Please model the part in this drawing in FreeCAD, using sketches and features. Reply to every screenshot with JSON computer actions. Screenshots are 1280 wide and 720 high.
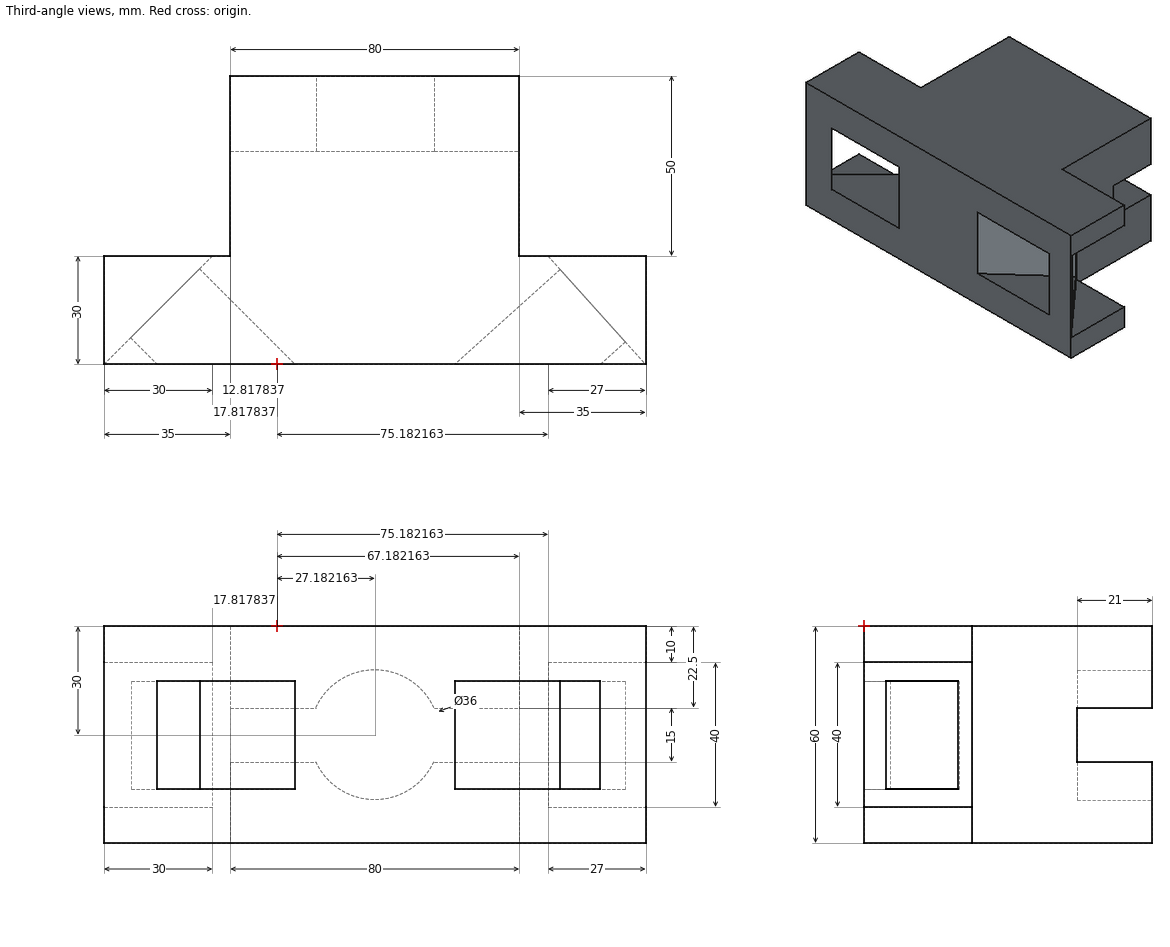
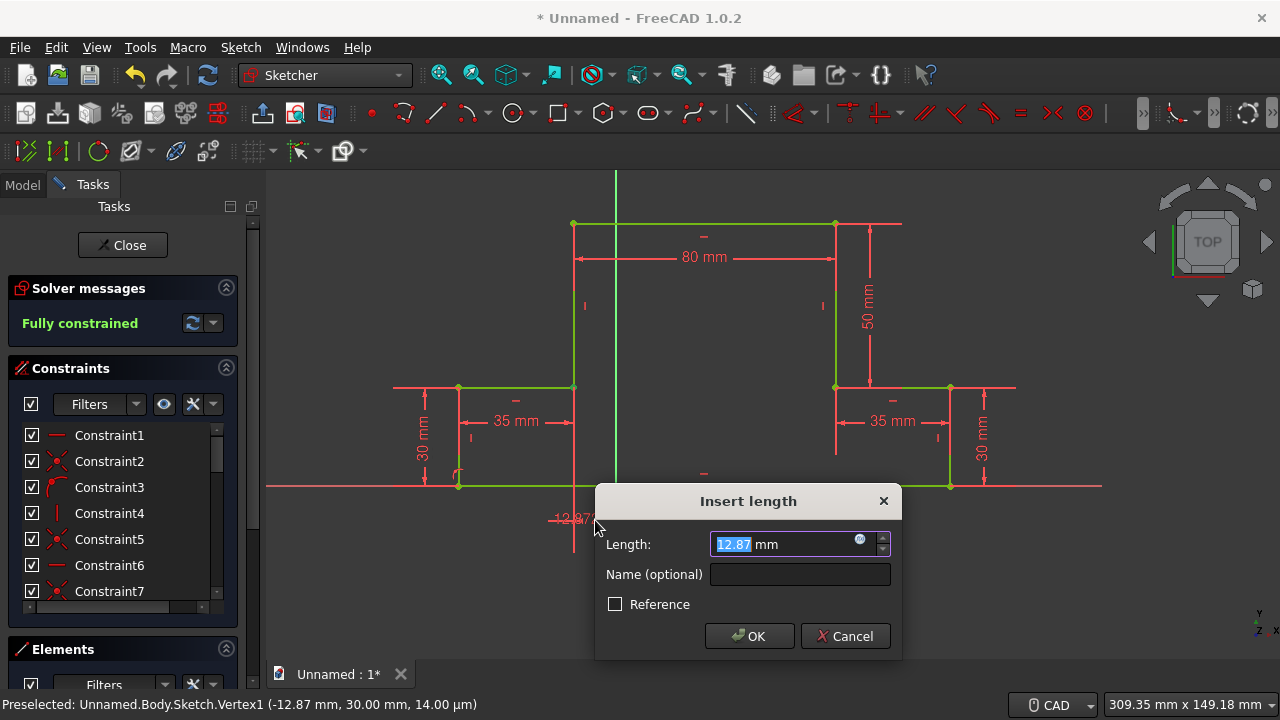
{"action": "type", "text": "12.817837"}
{"action": "key", "text": "Return"}
{"action": "key", "text": "Escape"}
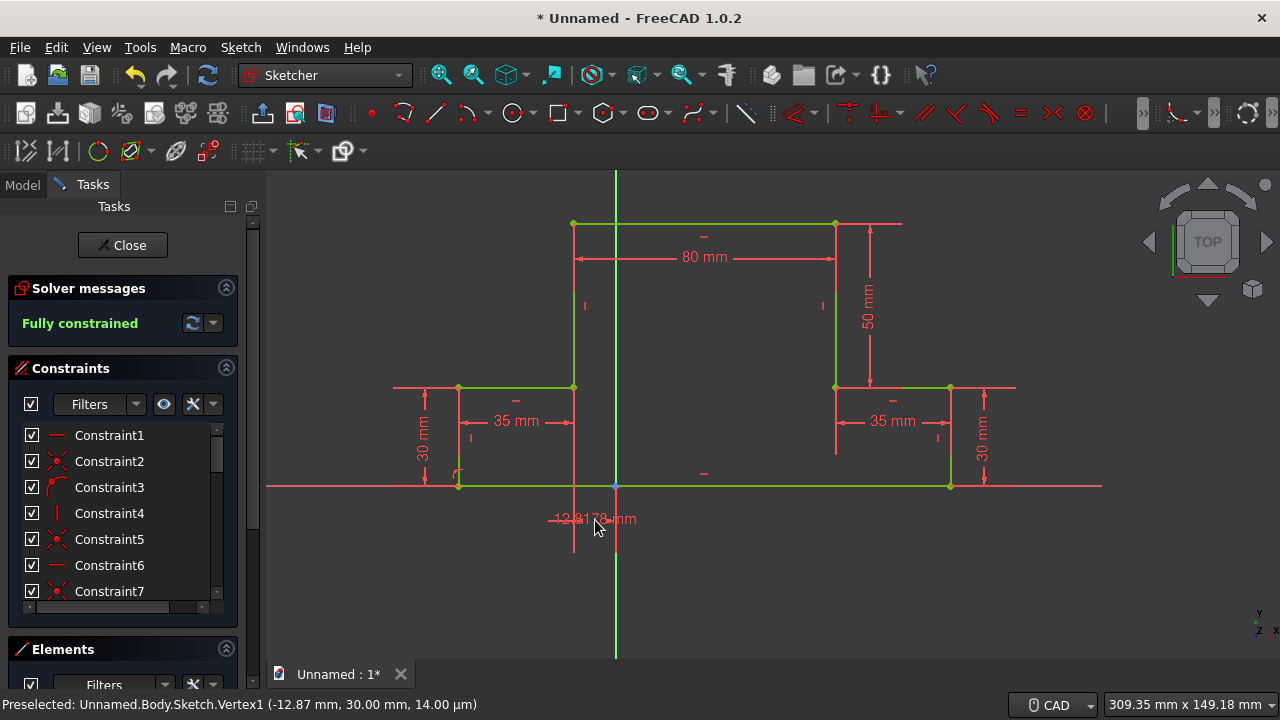
{"action": "left_click", "coordinate": [123, 245]}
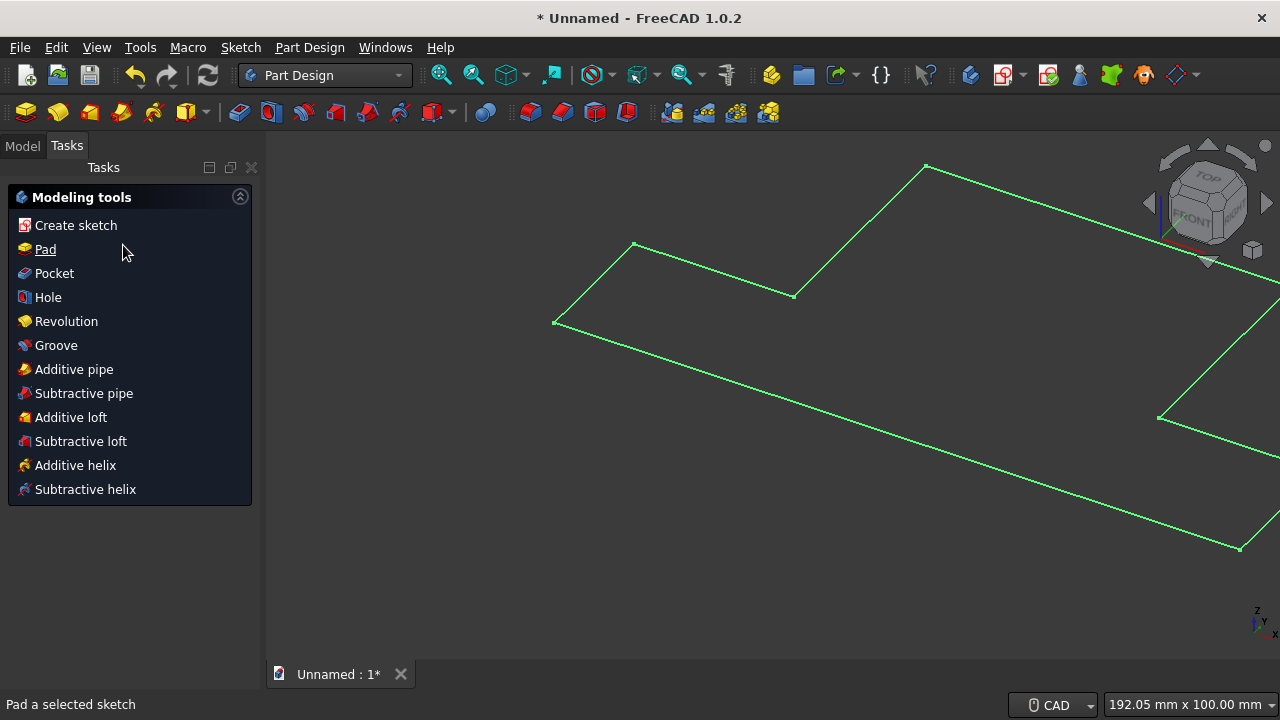
{"action": "left_click", "coordinate": [26, 112]}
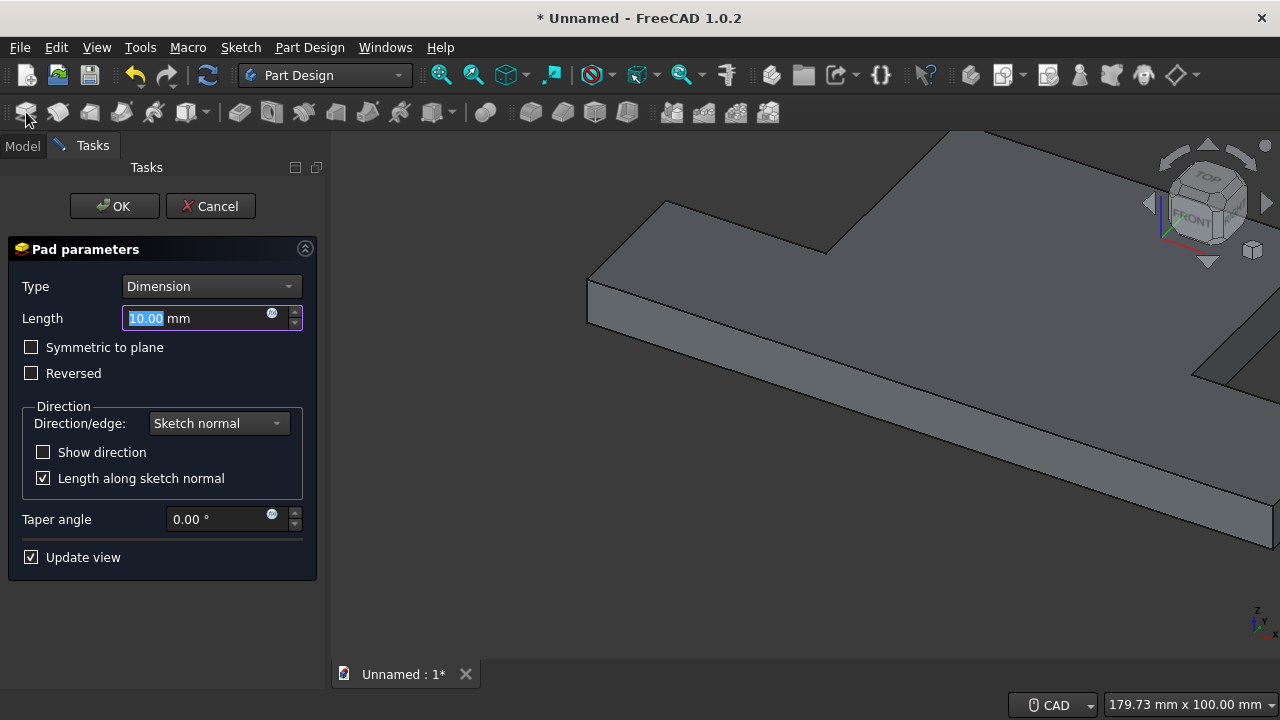
{"action": "type", "text": "60"}
{"action": "key", "text": "Tab"}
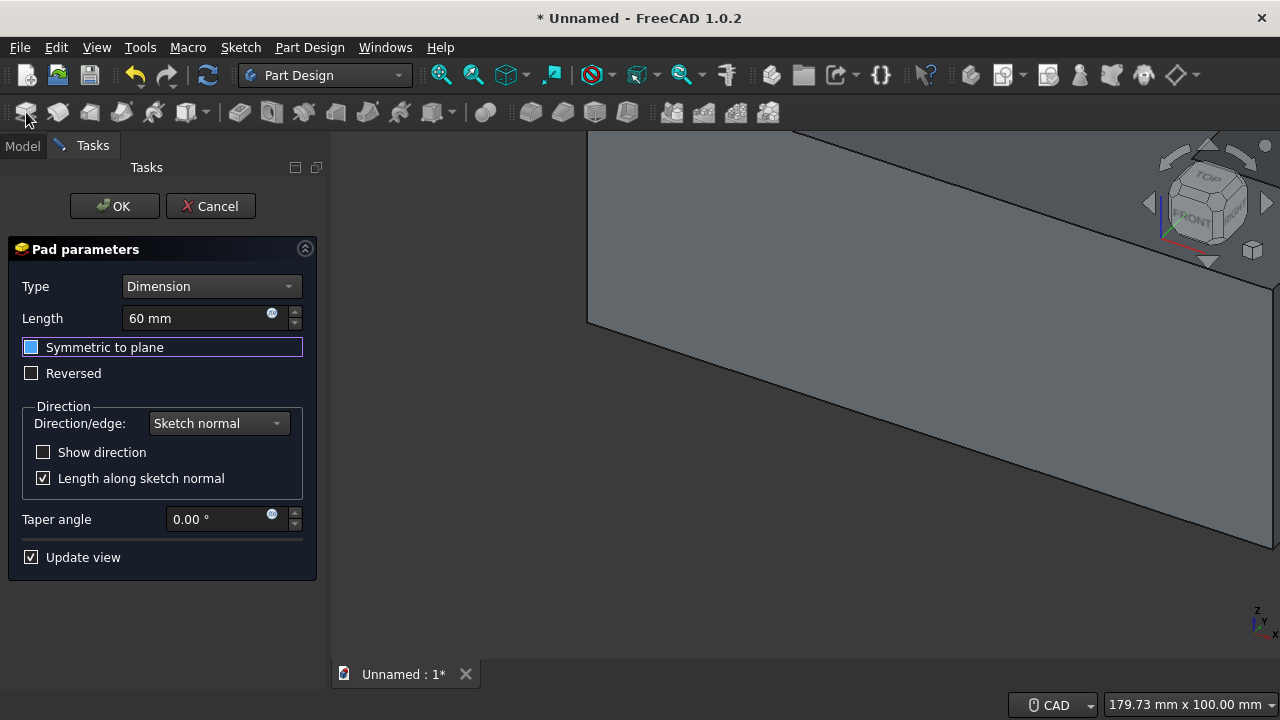
{"action": "left_click", "coordinate": [30, 373]}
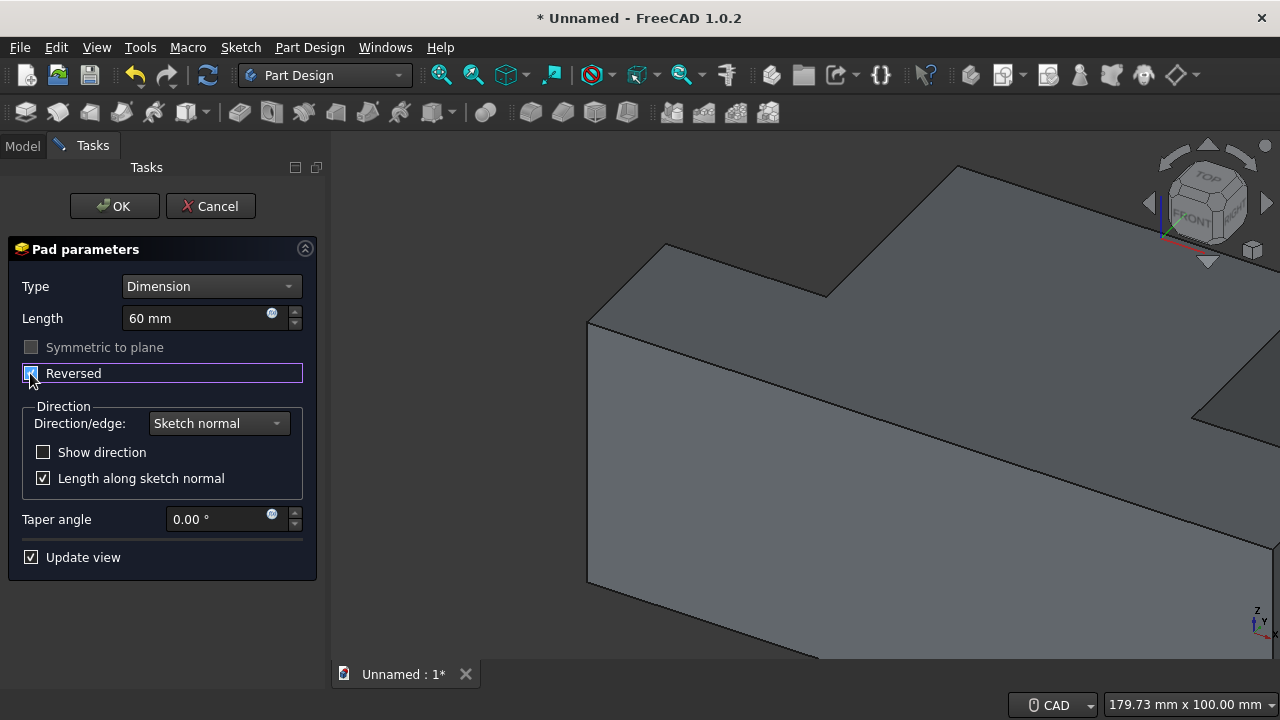
{"action": "left_click", "coordinate": [115, 206]}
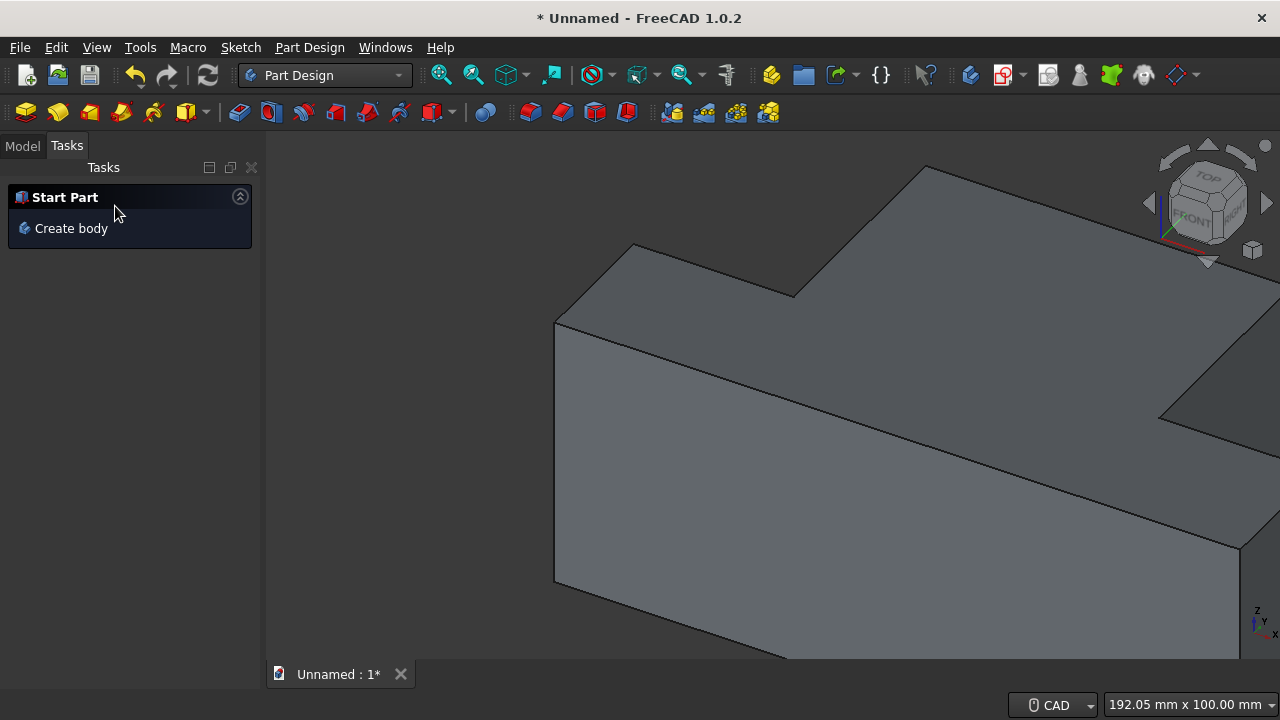
{"action": "left_click", "coordinate": [442, 76]}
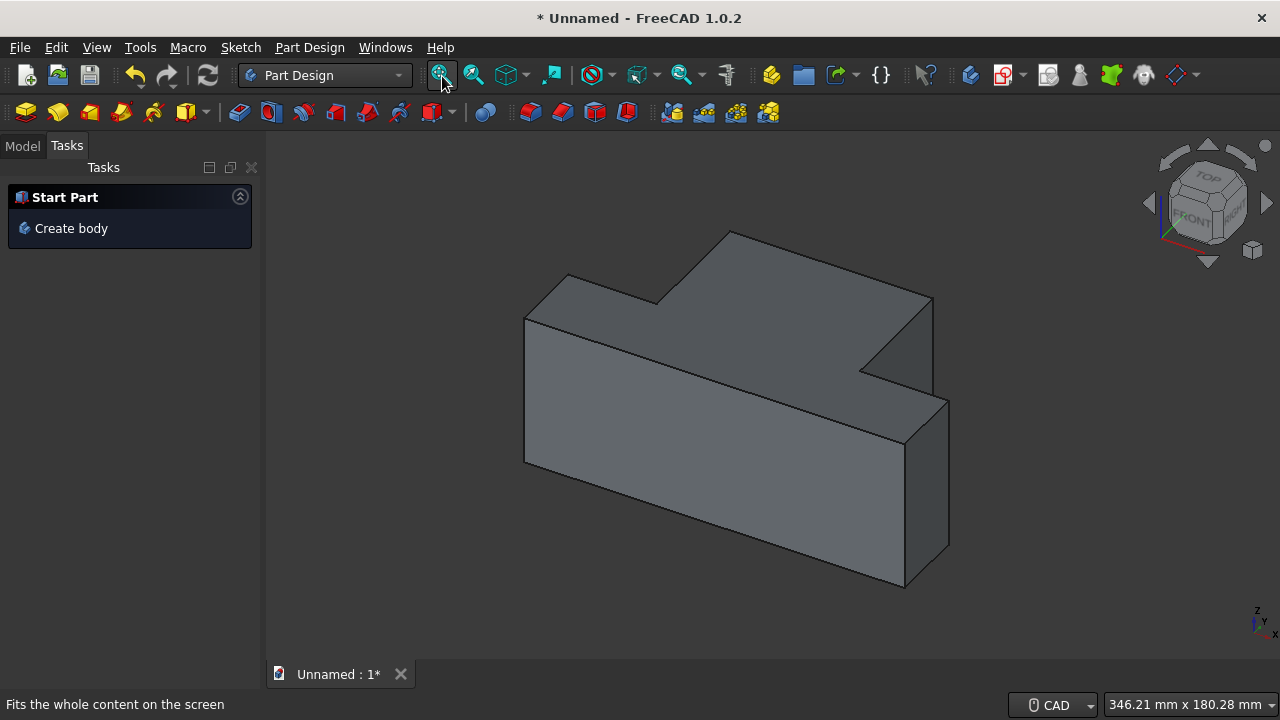
{"action": "key", "text": "4"}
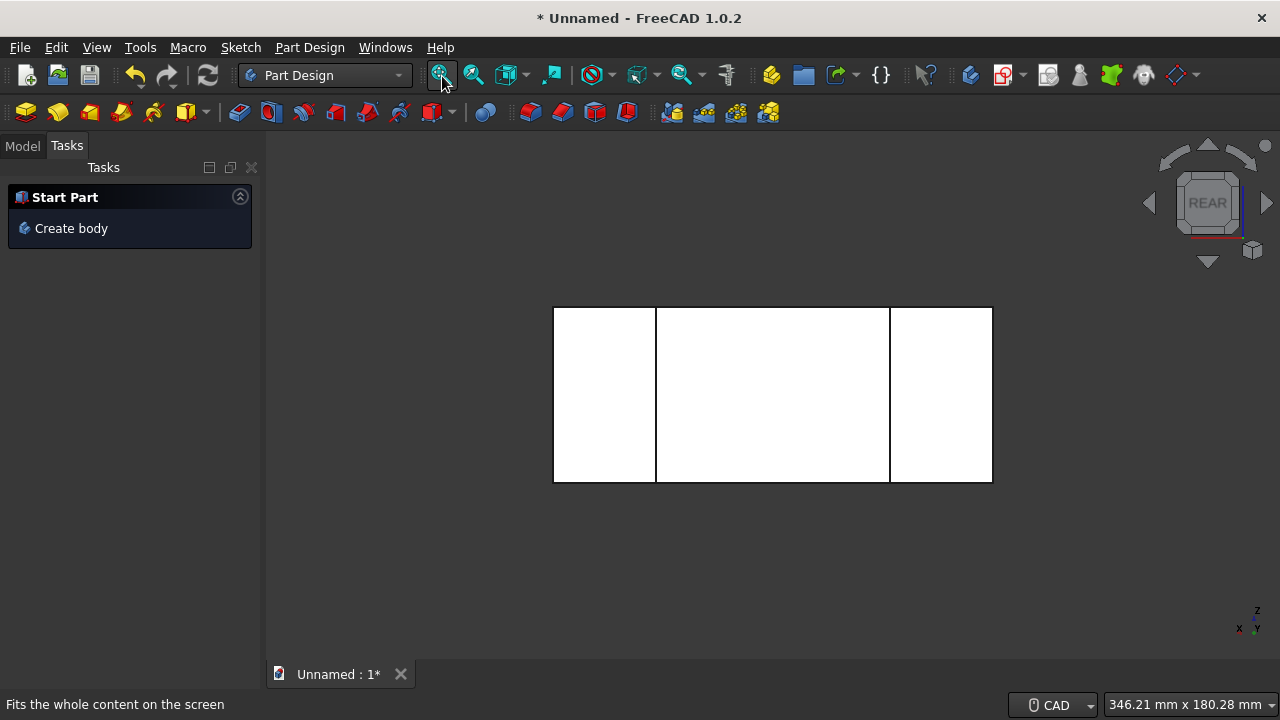
{"action": "left_click", "coordinate": [442, 76]}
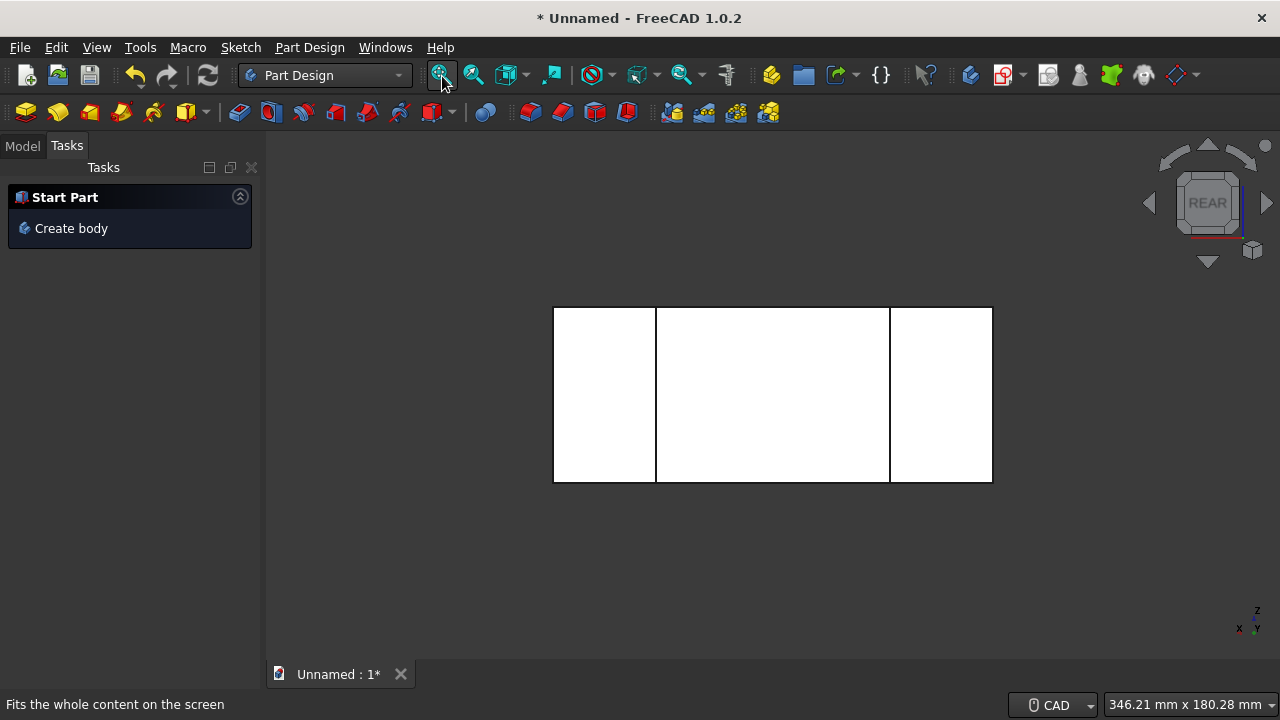
{"action": "left_click", "coordinate": [773, 394]}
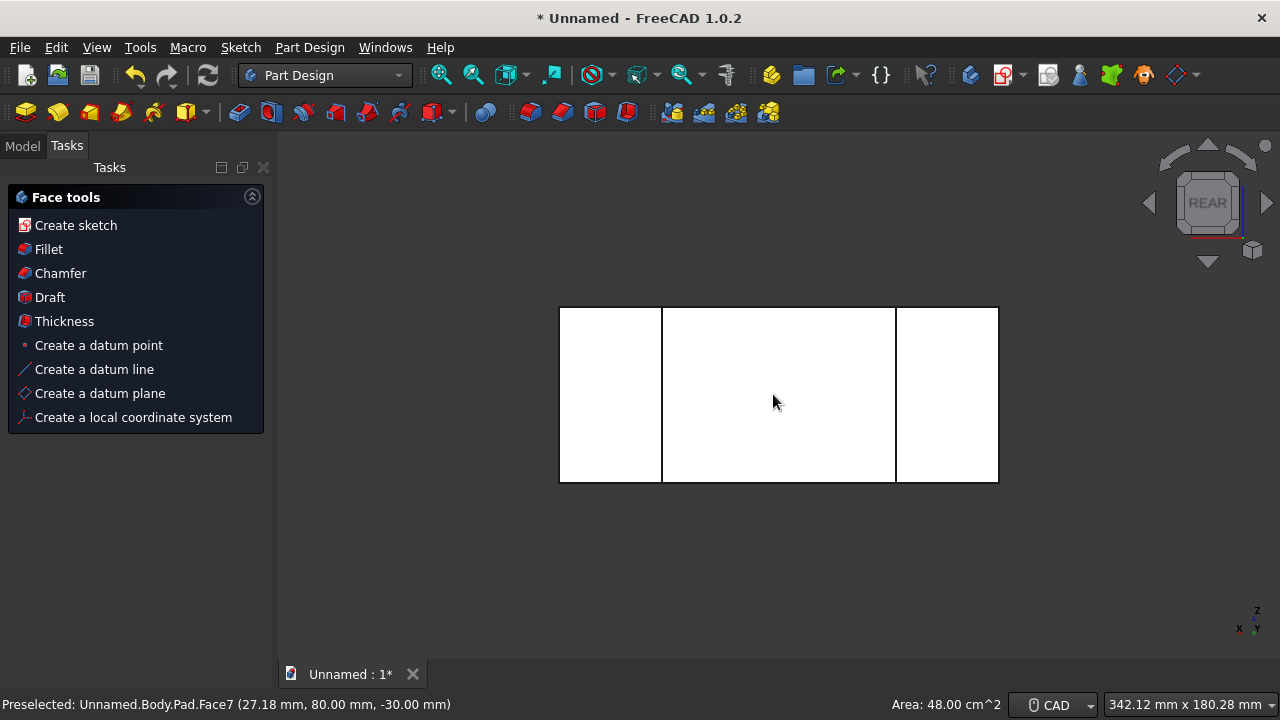
{"action": "left_click", "coordinate": [1004, 76]}